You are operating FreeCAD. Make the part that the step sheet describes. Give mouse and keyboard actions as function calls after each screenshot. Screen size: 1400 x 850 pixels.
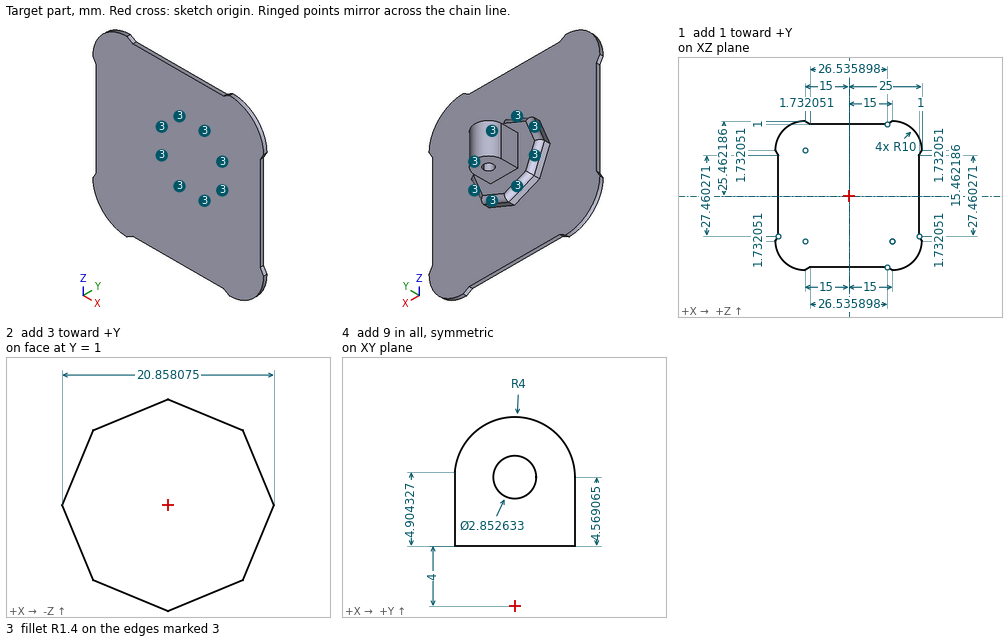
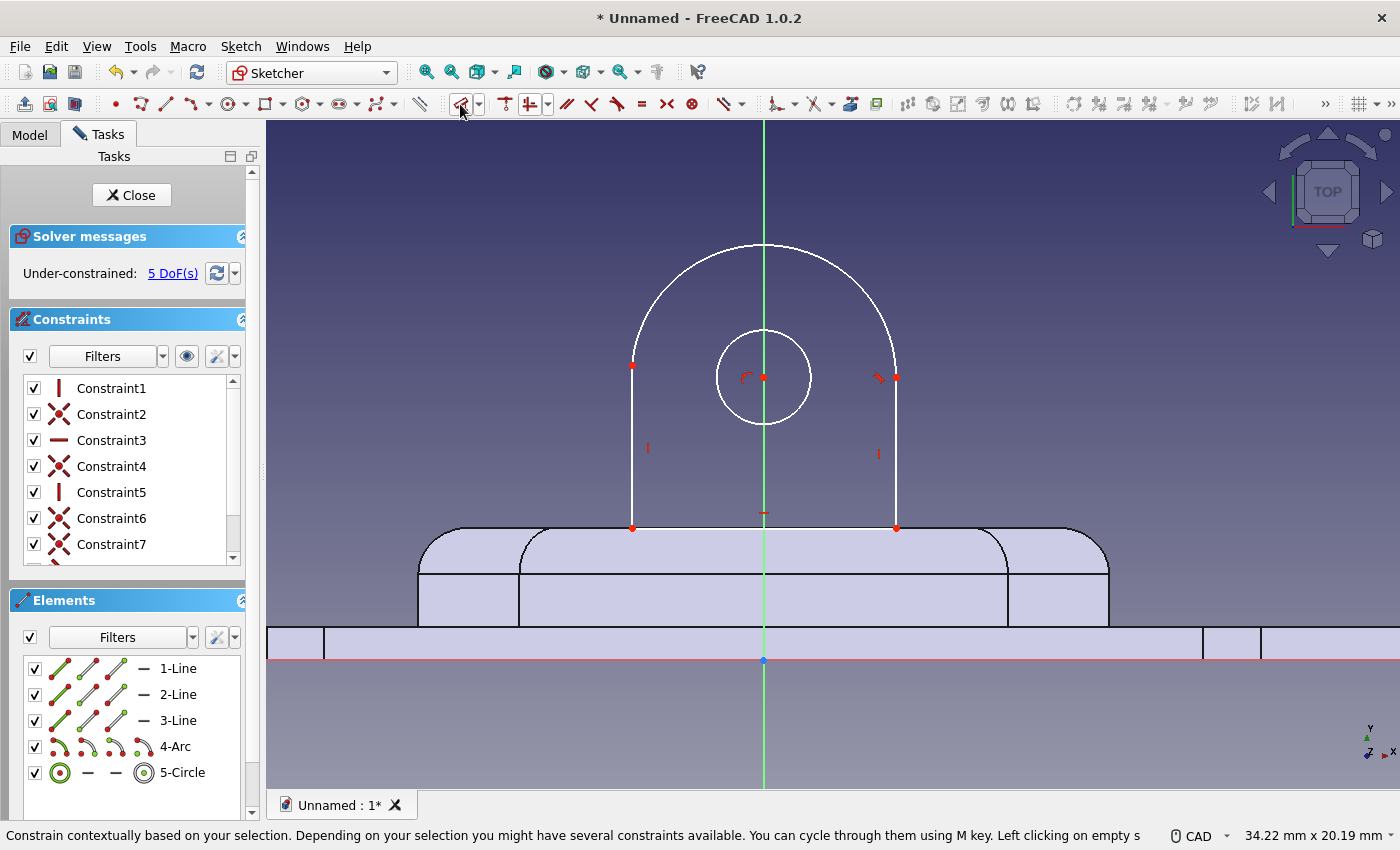
click(844, 272)
click(863, 247)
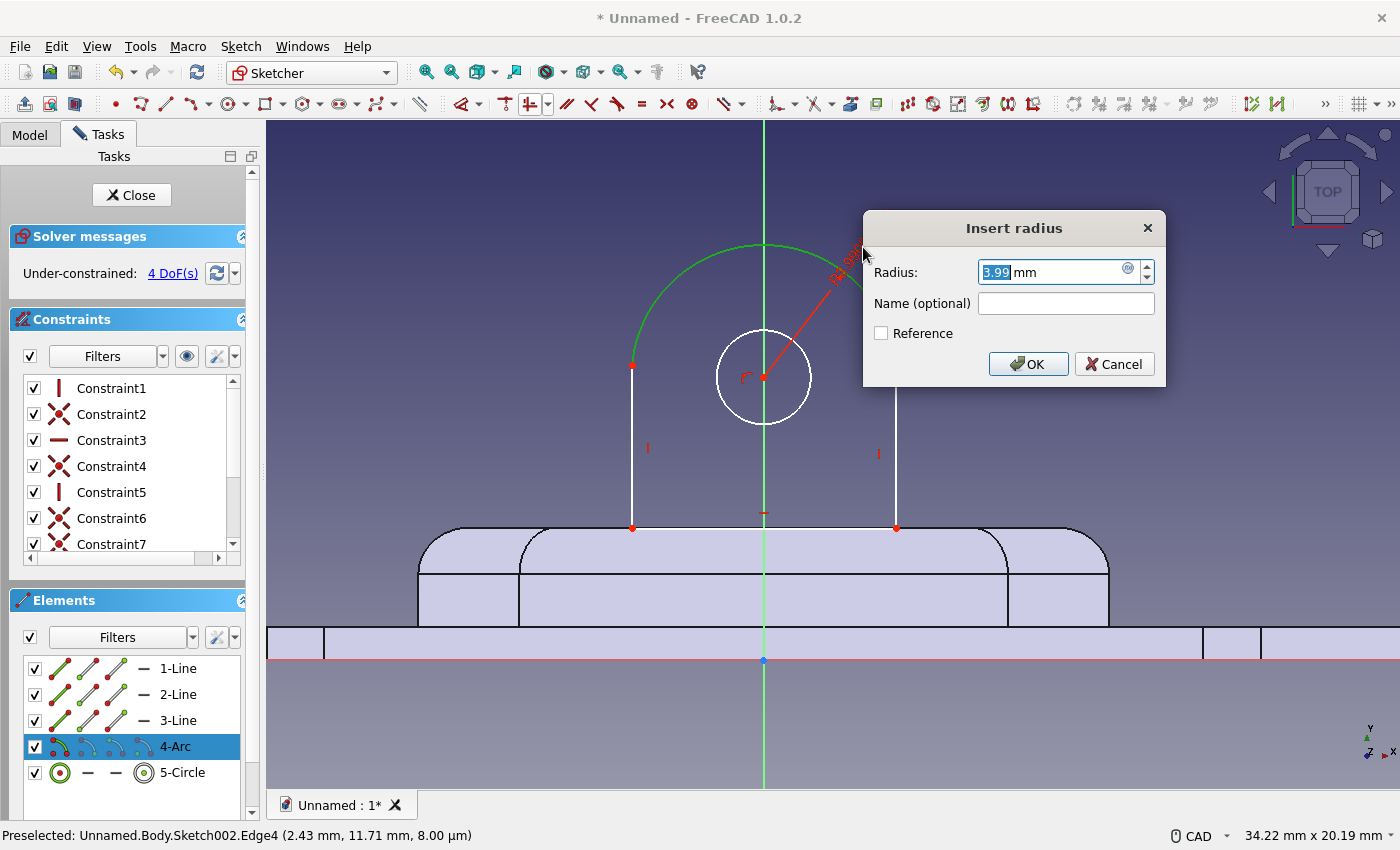
text(4)
key(Return)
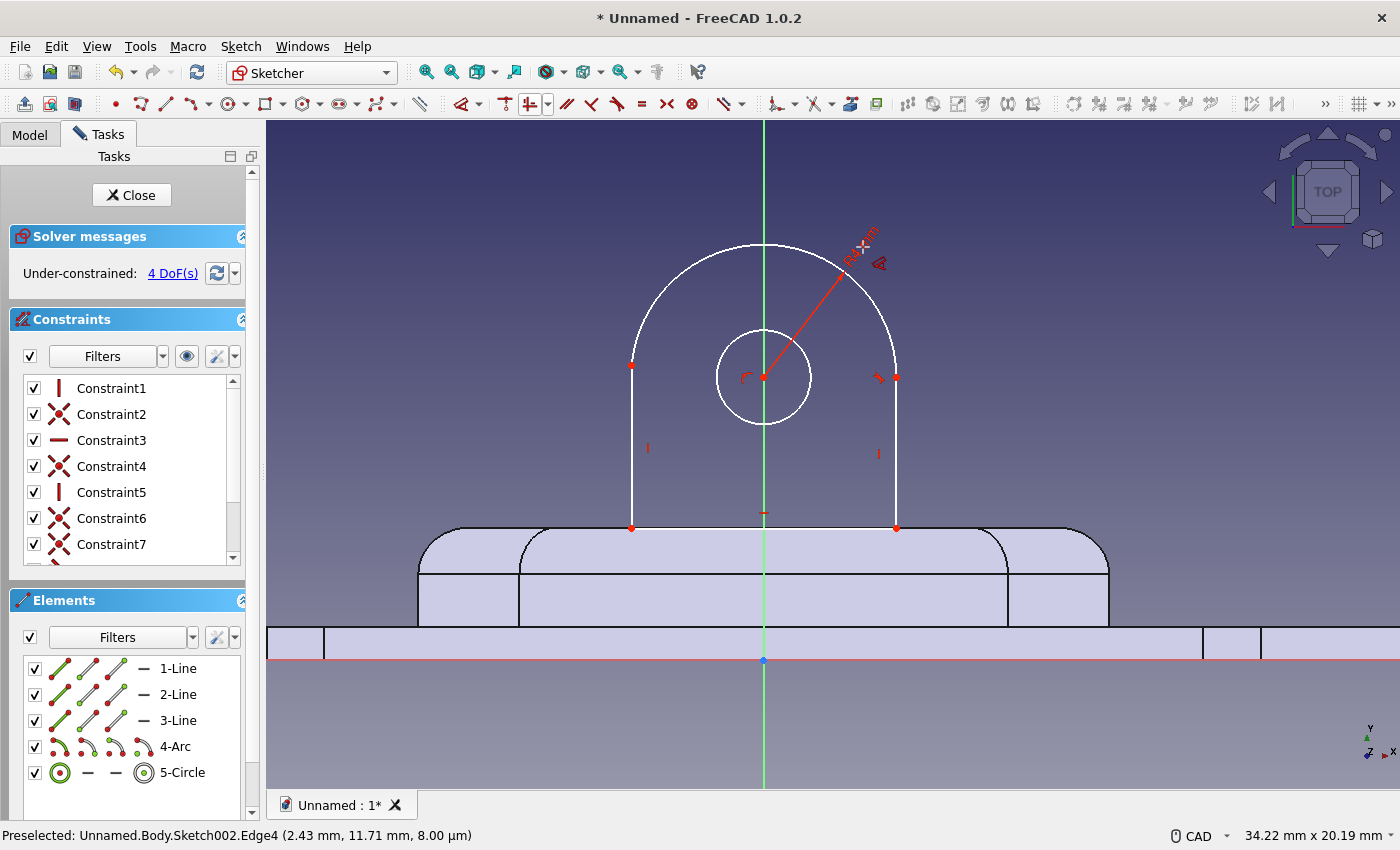
click(797, 344)
click(820, 321)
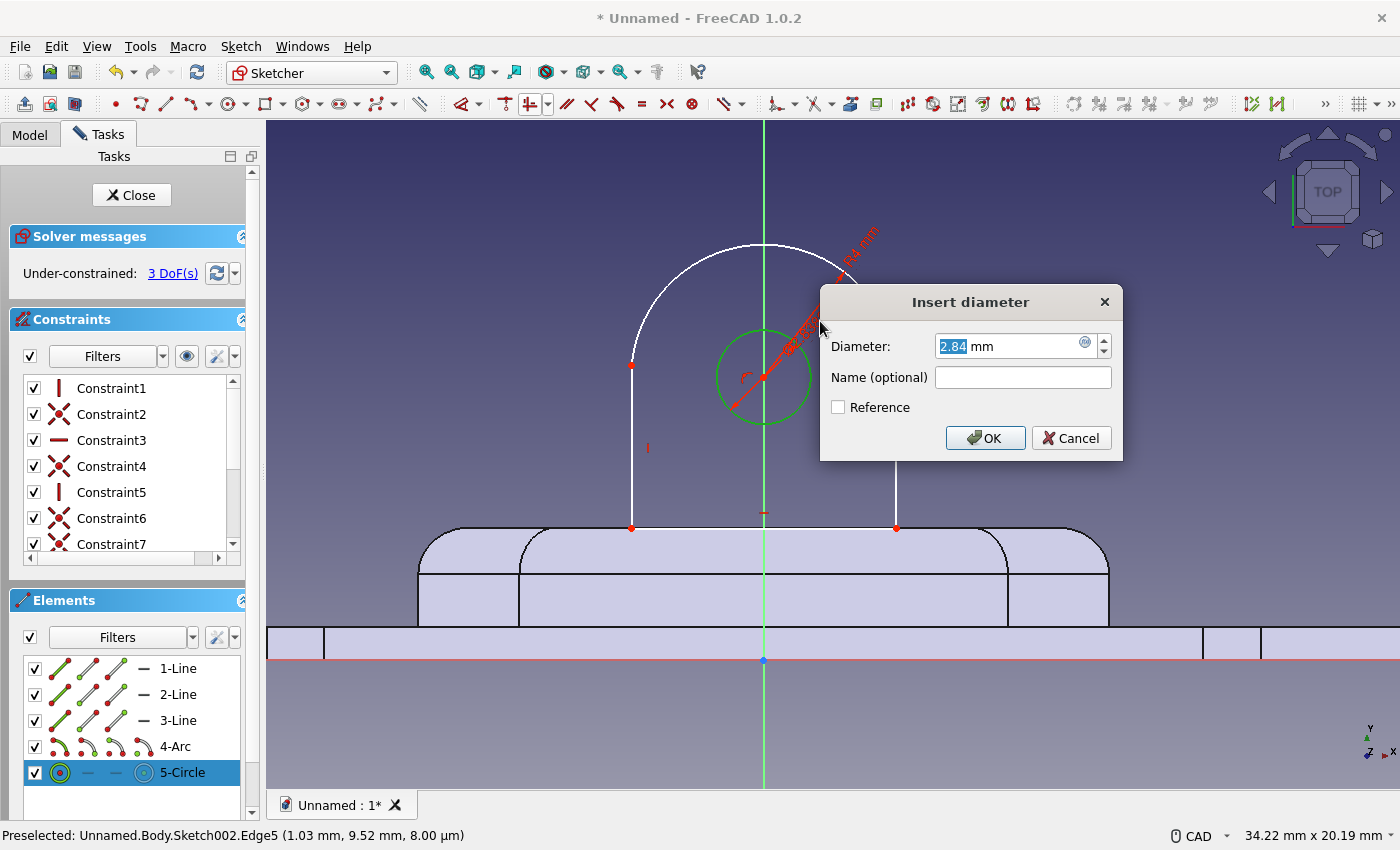
text(2.852633)
key(Return)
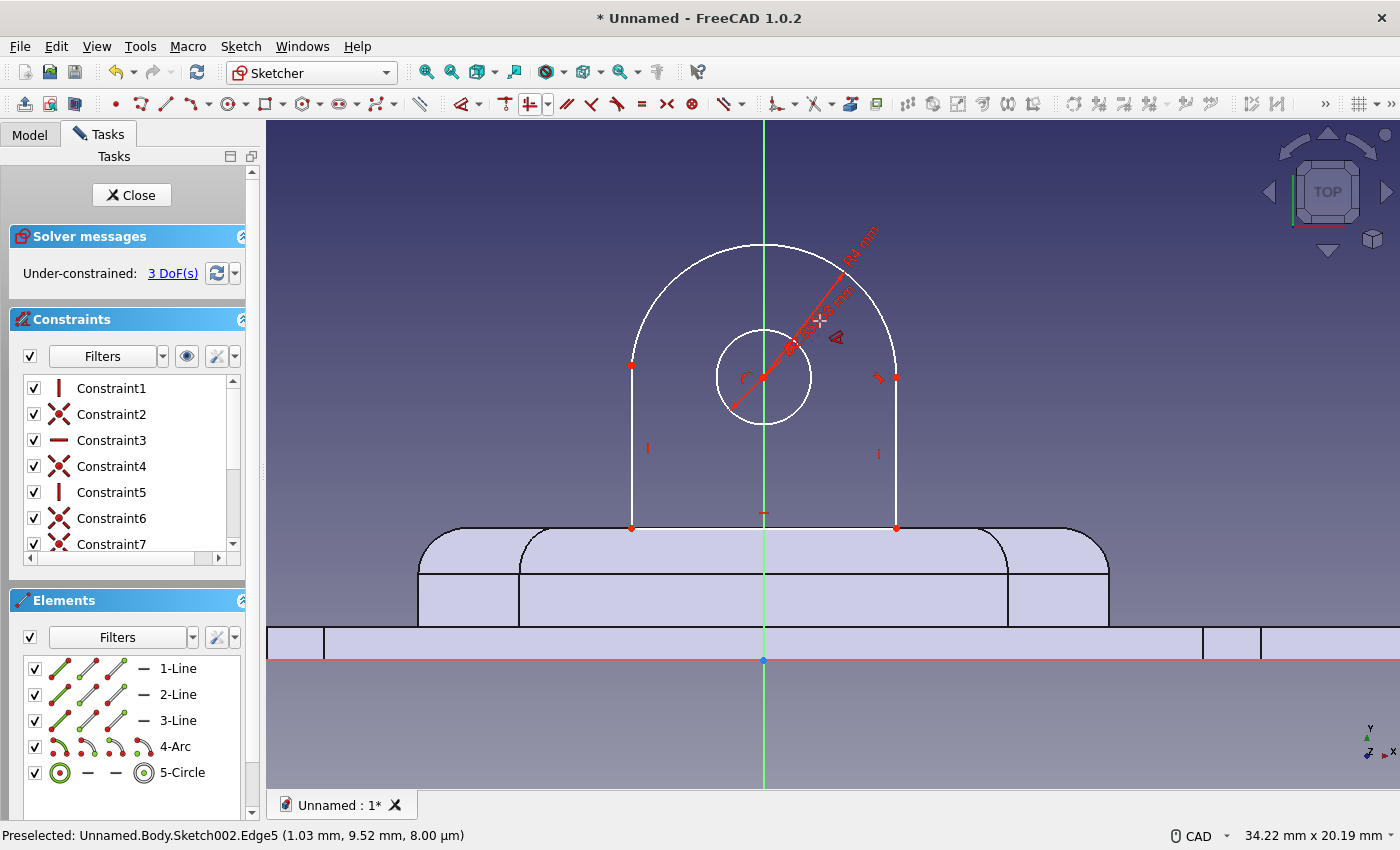
click(632, 529)
click(598, 595)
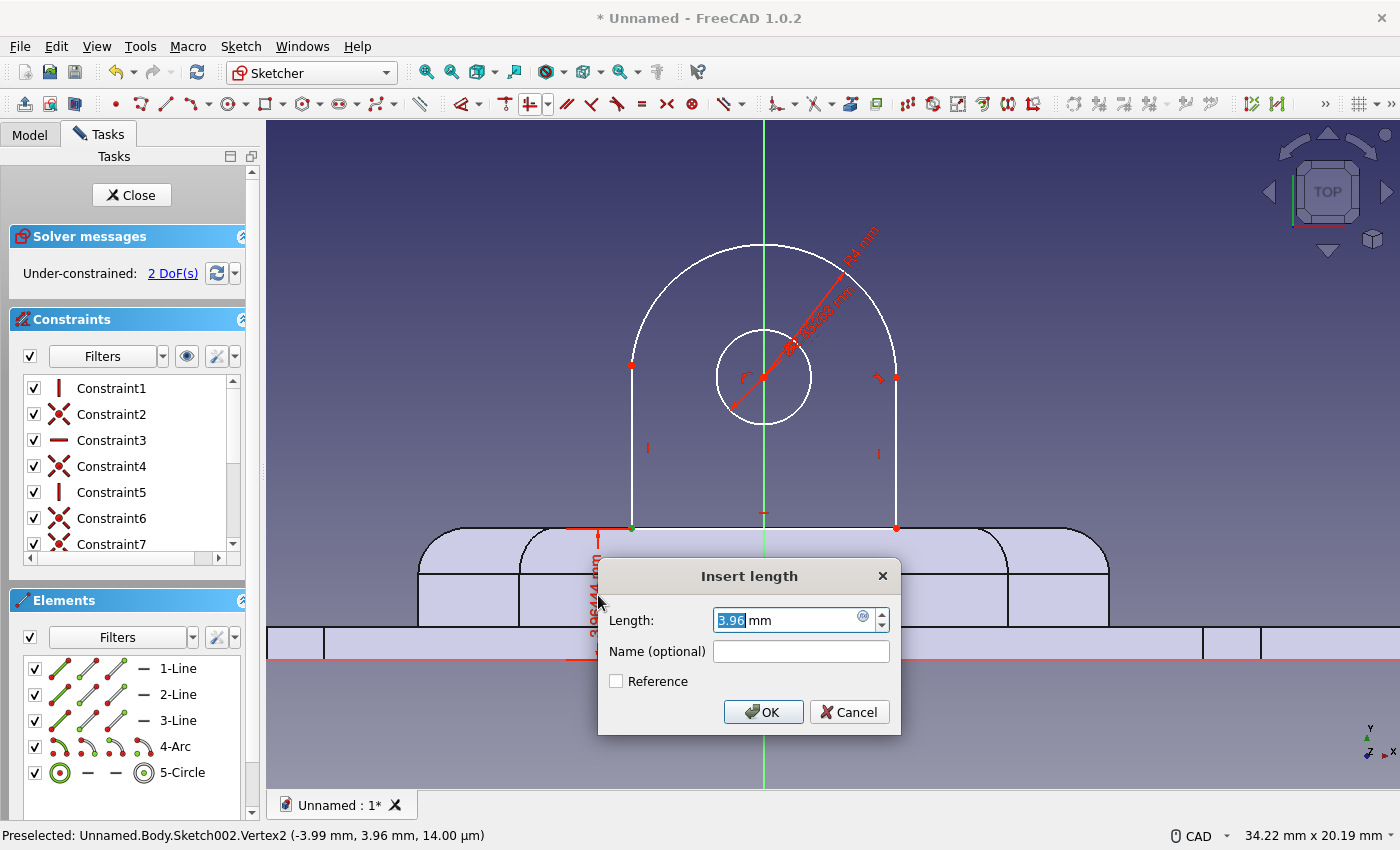
text(4)
key(Return)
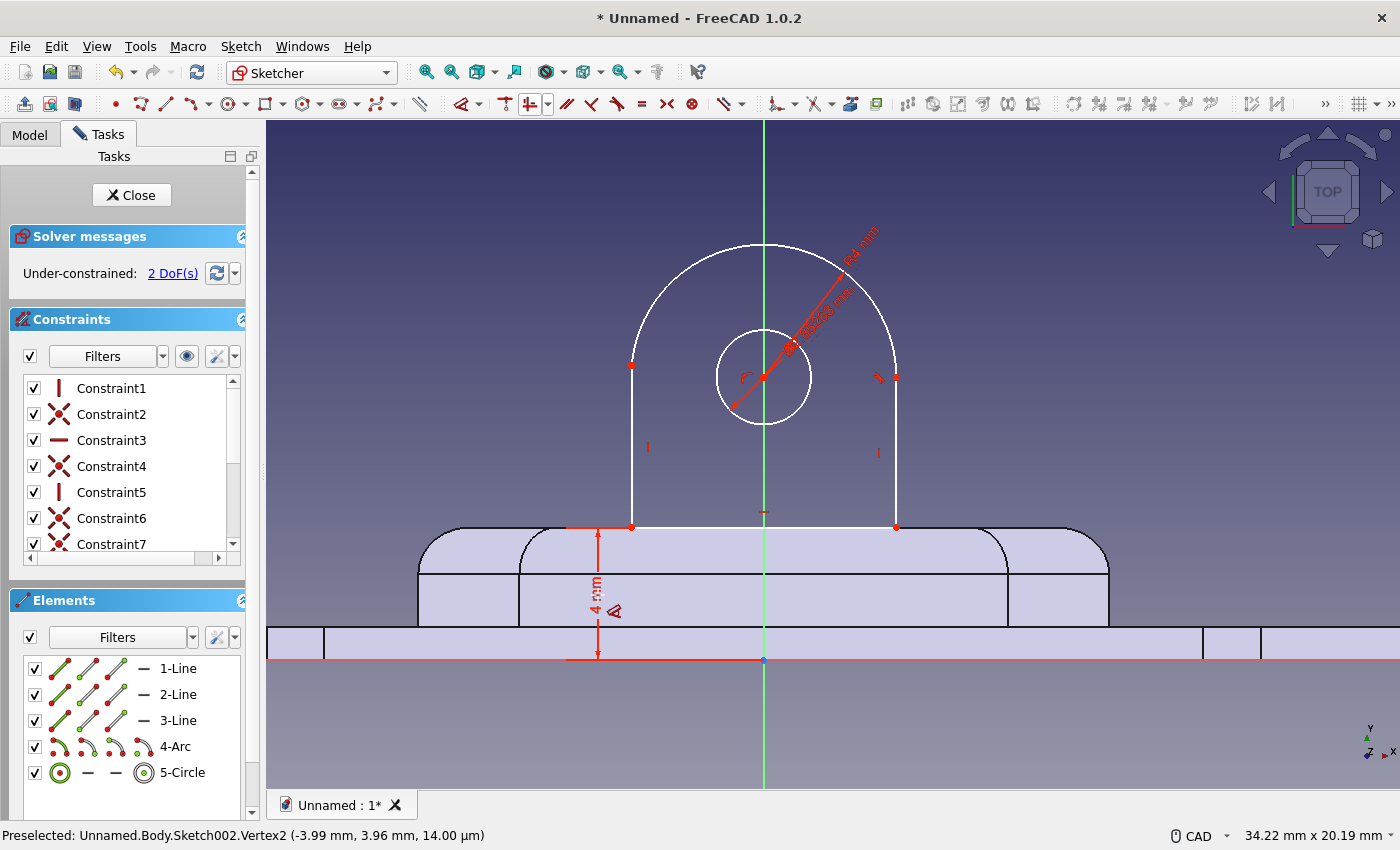
click(632, 415)
click(598, 447)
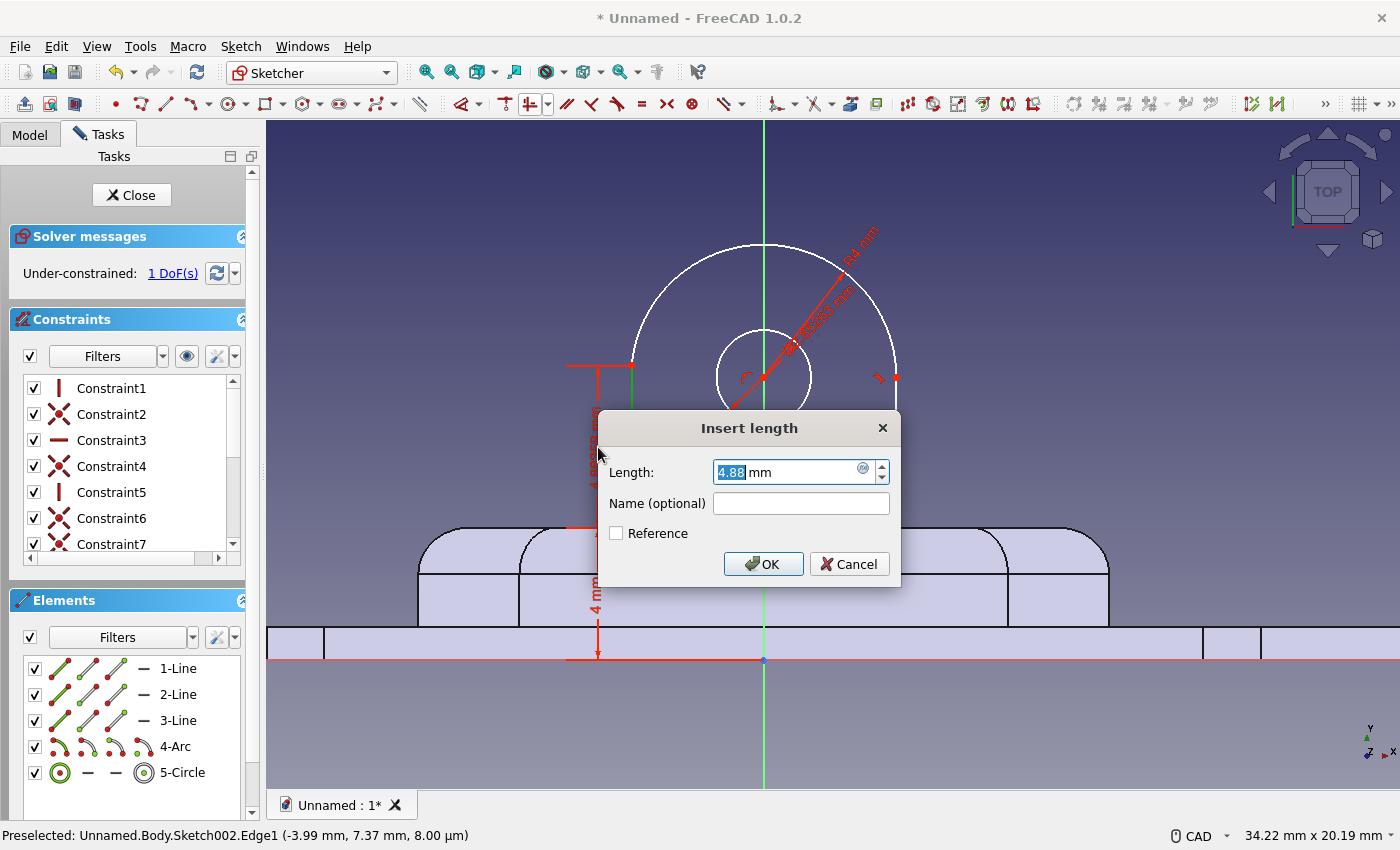
text(4.904327)
key(Return)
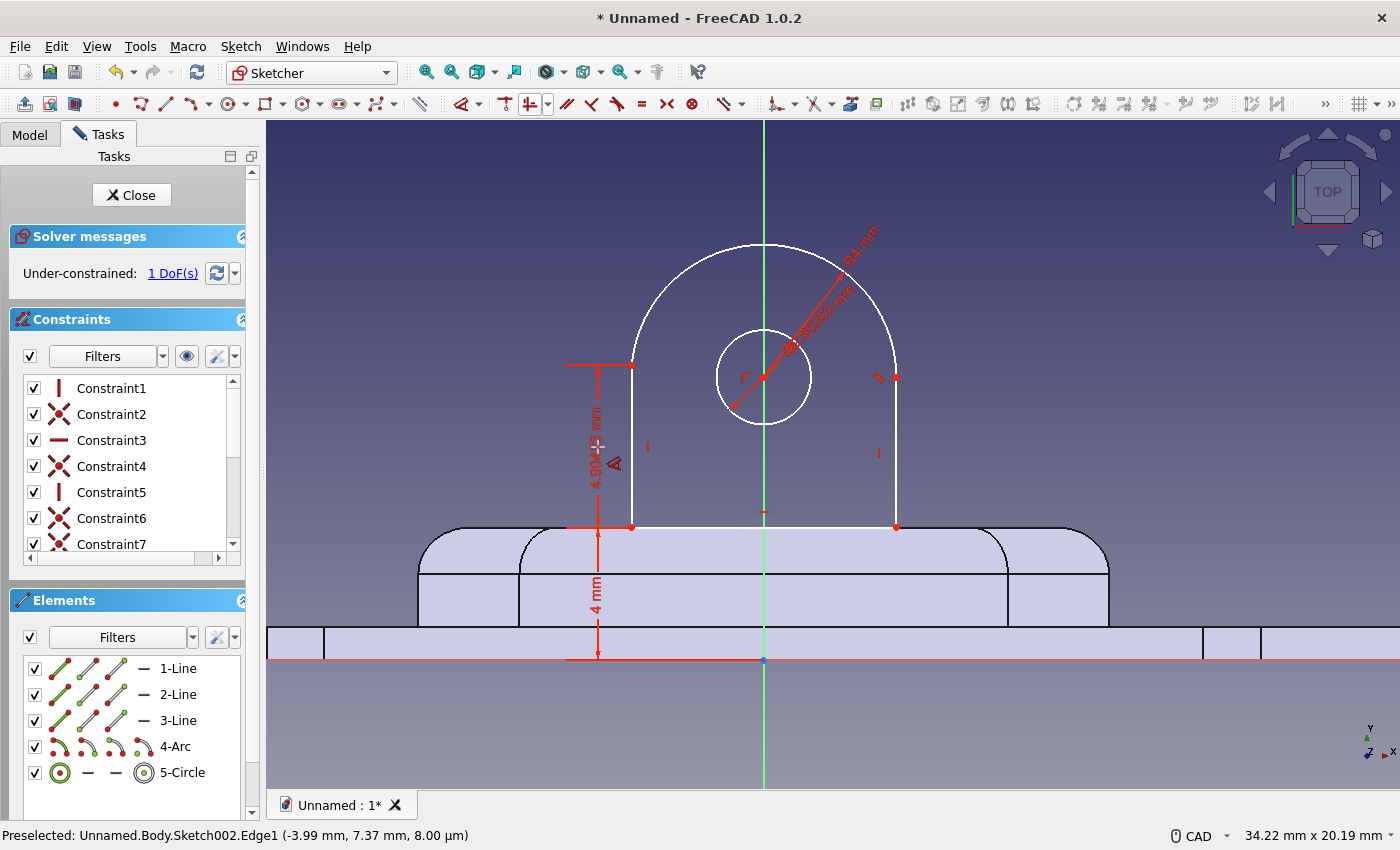
click(896, 483)
click(930, 453)